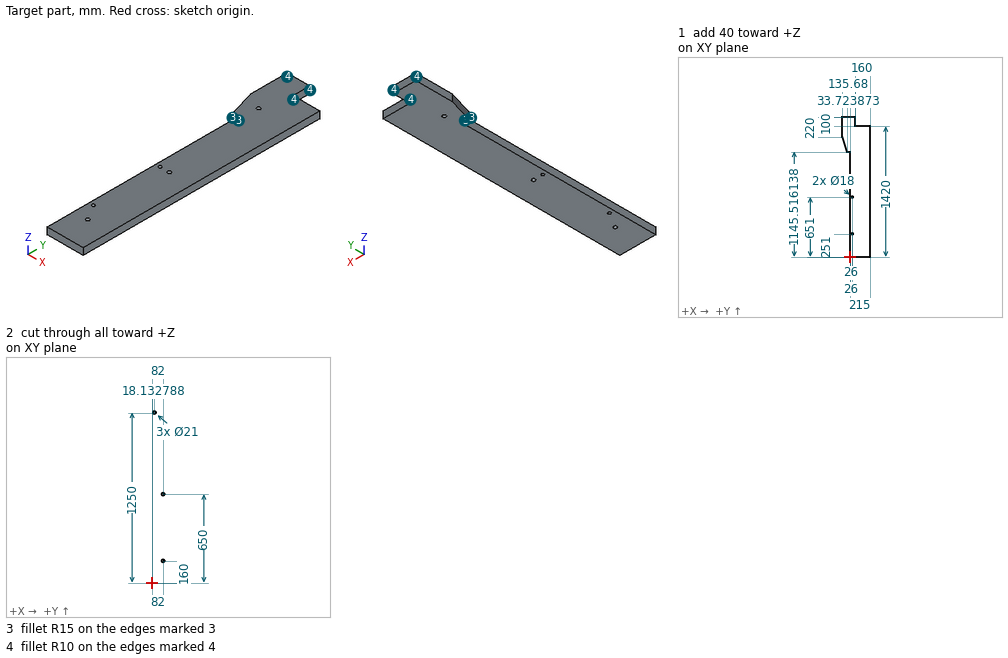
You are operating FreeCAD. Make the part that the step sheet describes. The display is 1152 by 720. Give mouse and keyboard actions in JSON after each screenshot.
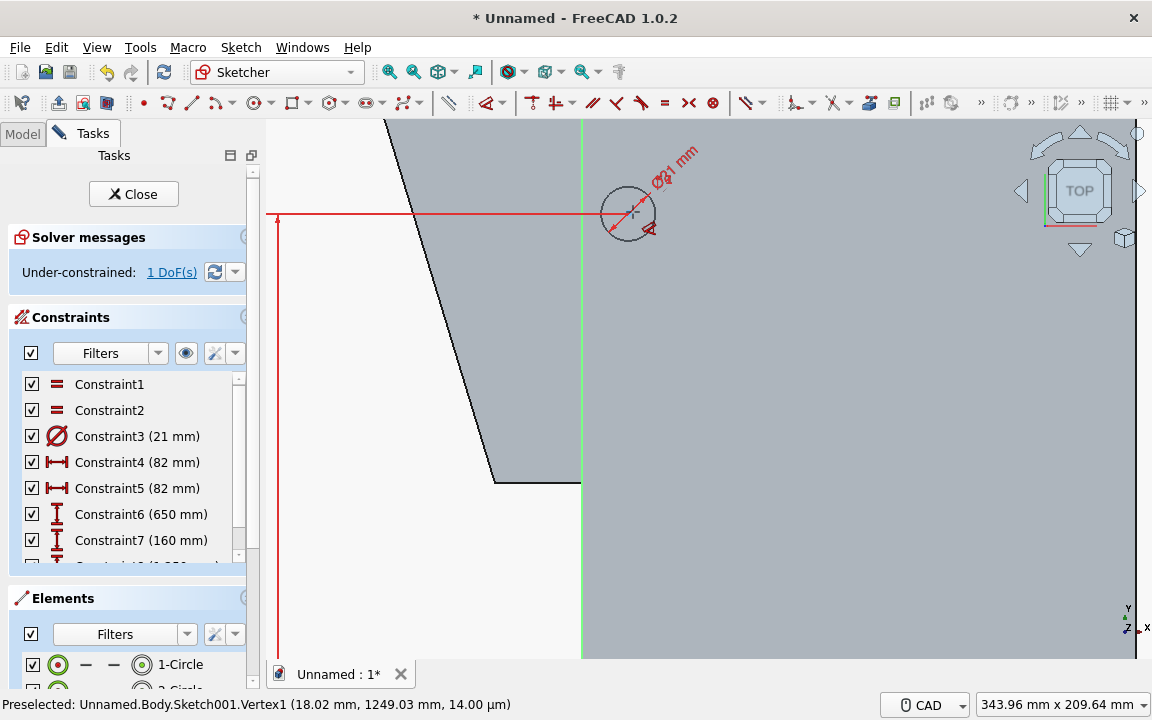
{"action": "left_click", "coordinate": [628, 214]}
{"action": "left_click", "coordinate": [605, 180]}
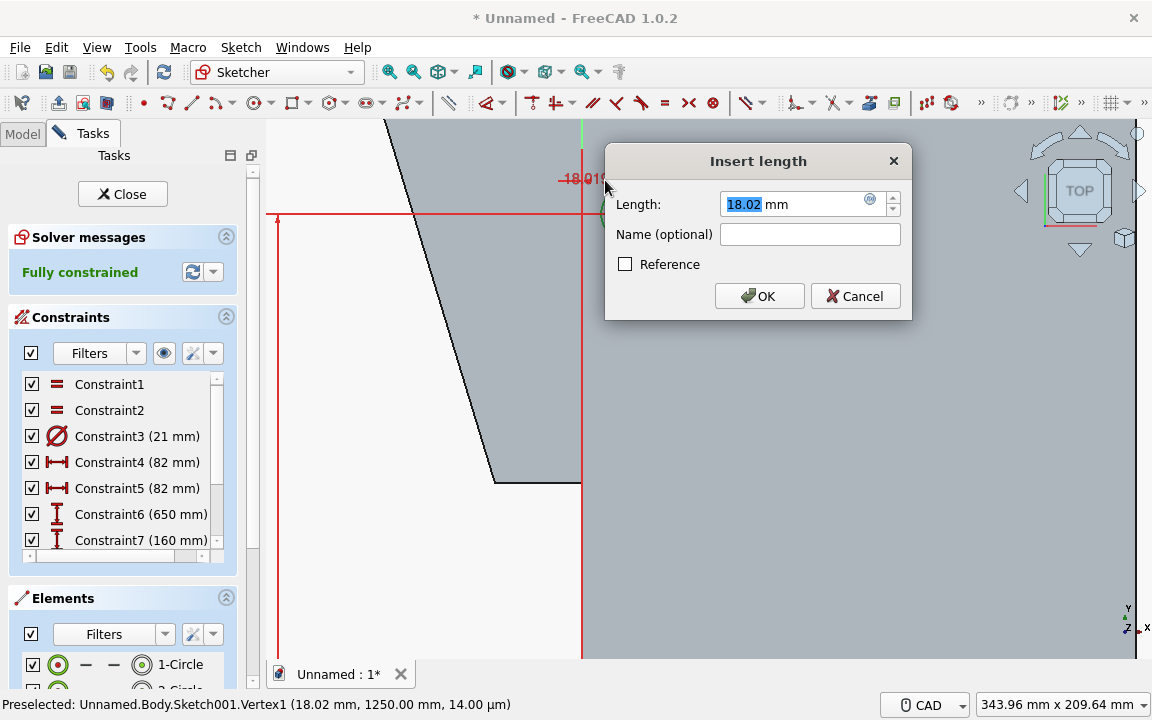
{"action": "type", "text": "18.132788"}
{"action": "key", "text": "Return"}
{"action": "key", "text": "Escape"}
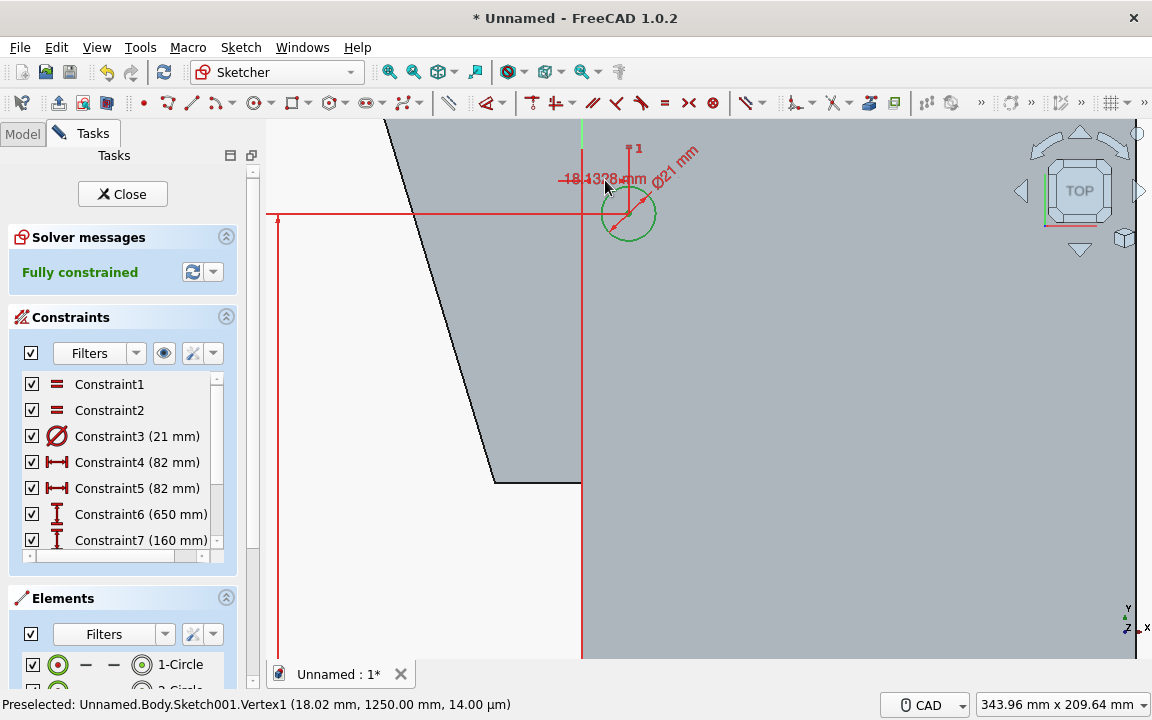
{"action": "left_click", "coordinate": [123, 194]}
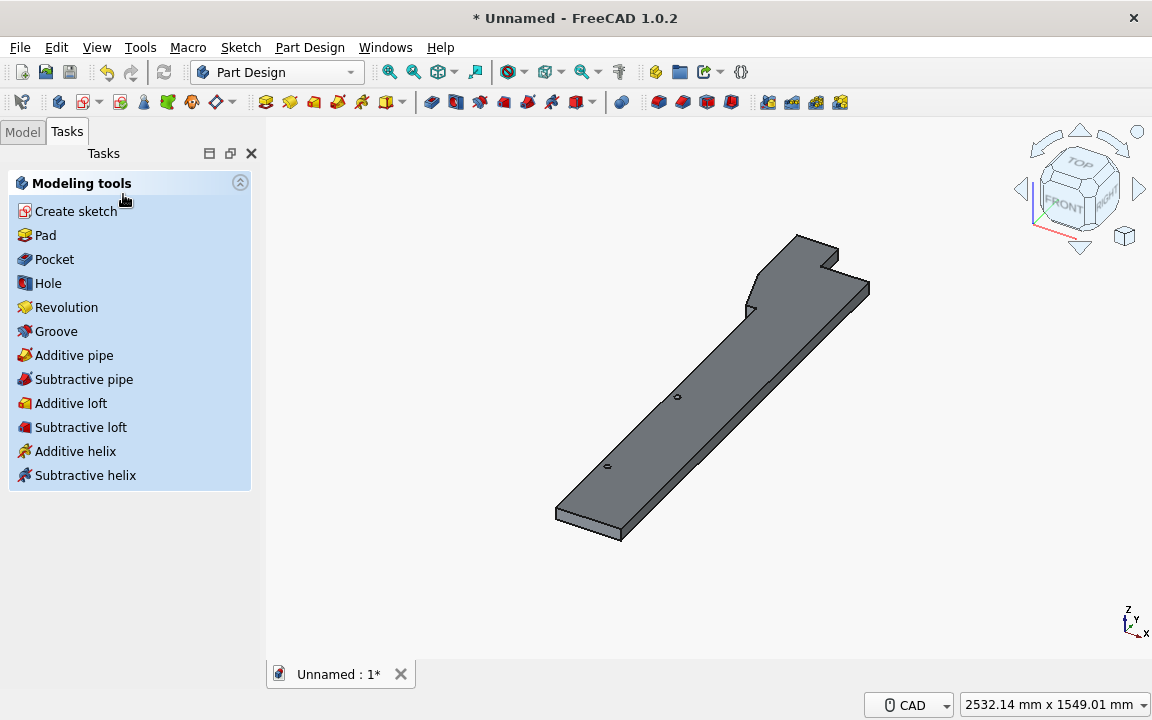
{"action": "left_click", "coordinate": [432, 102]}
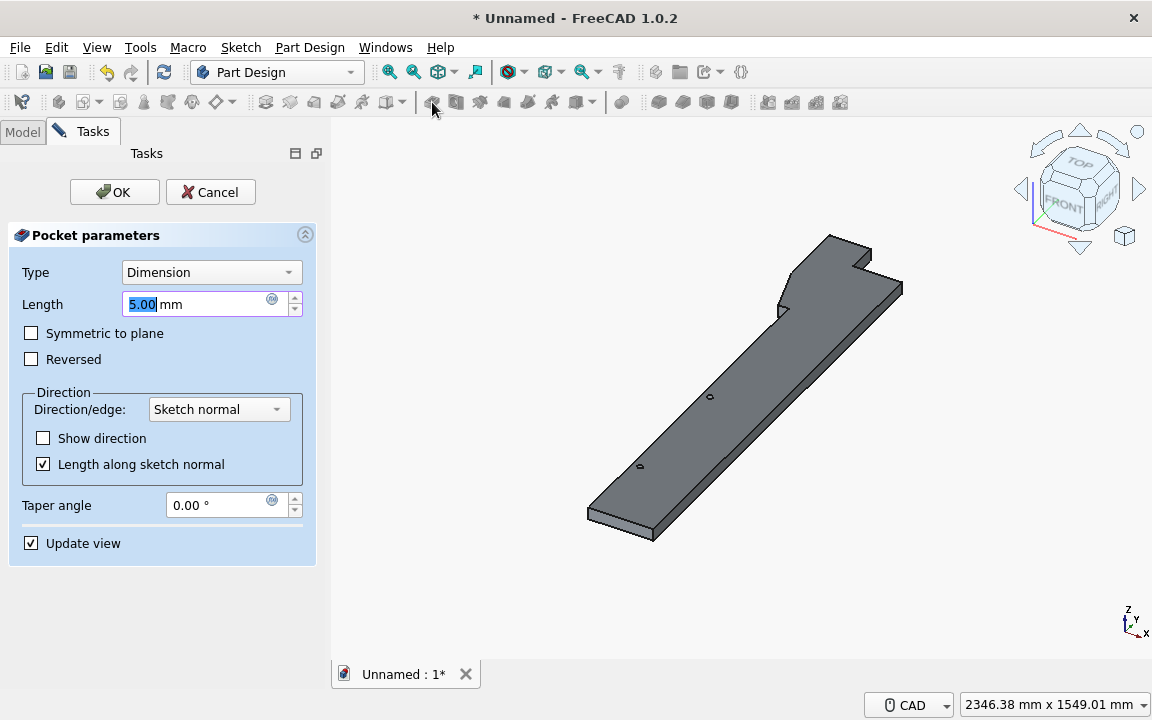
{"action": "left_click", "coordinate": [212, 272]}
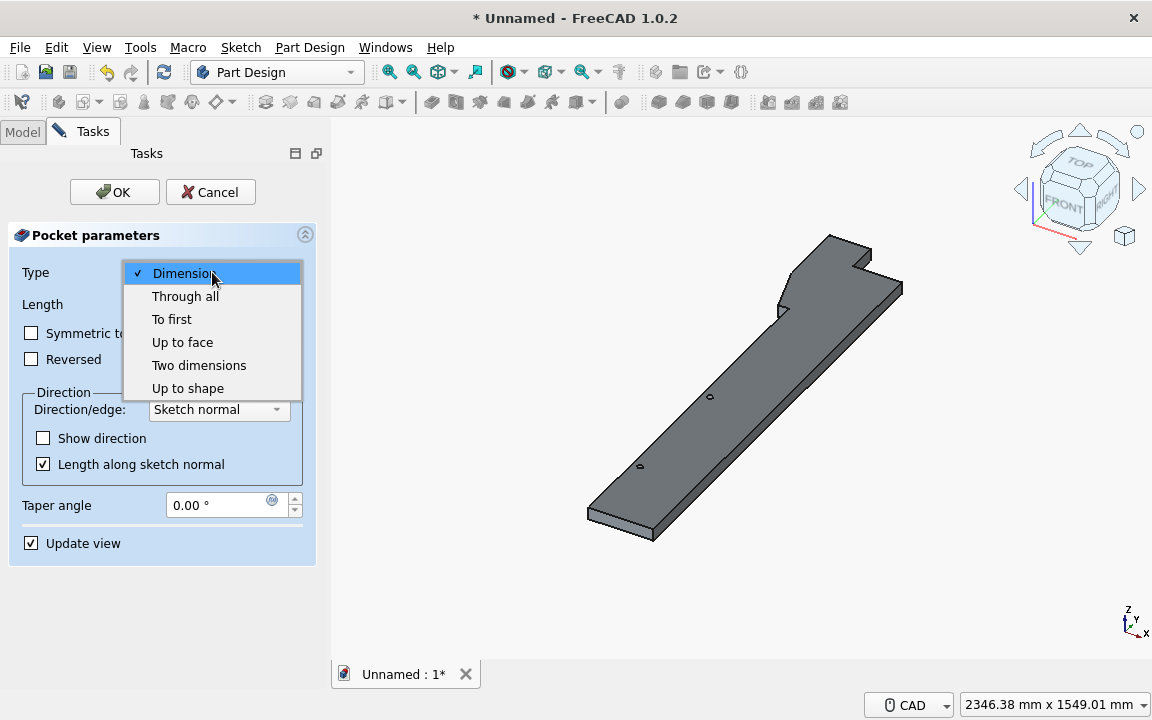
{"action": "left_click", "coordinate": [212, 296]}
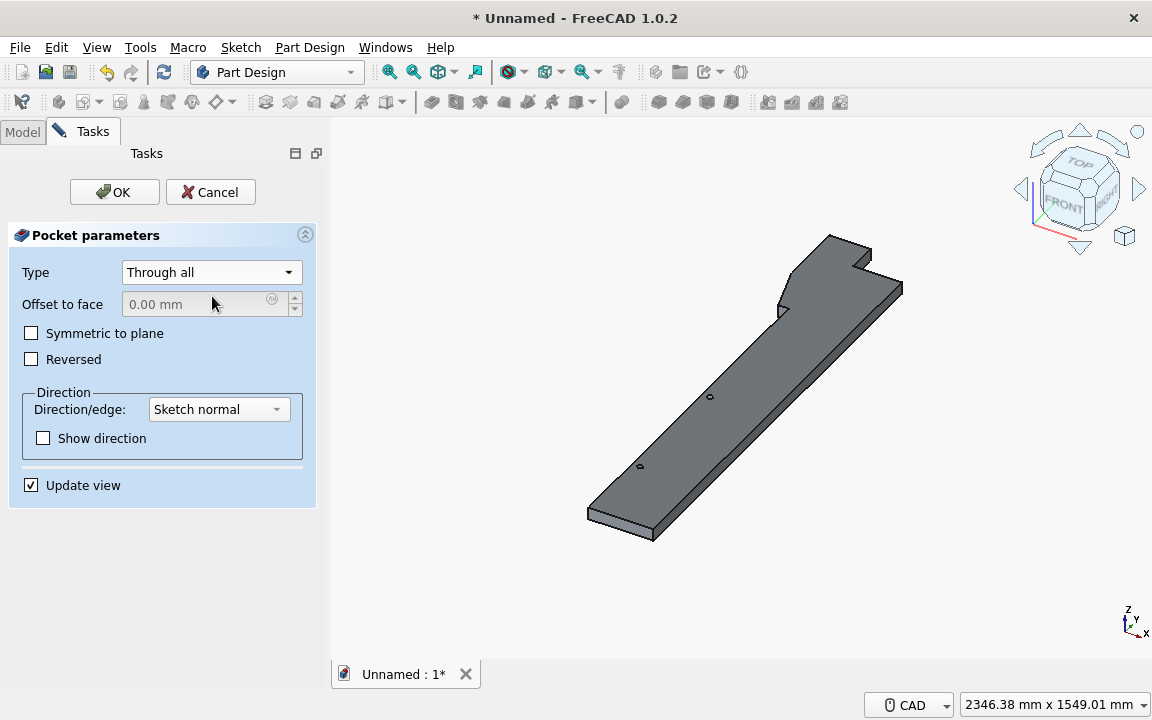
{"action": "left_click", "coordinate": [30, 359]}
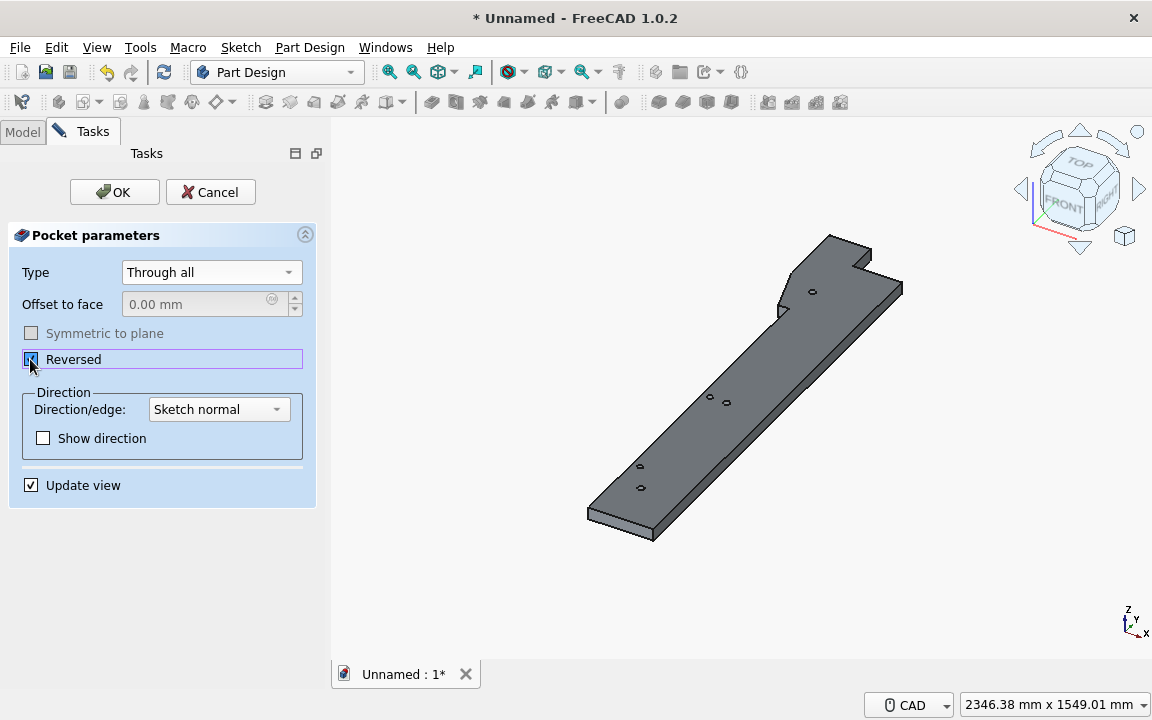
{"action": "left_click", "coordinate": [115, 192]}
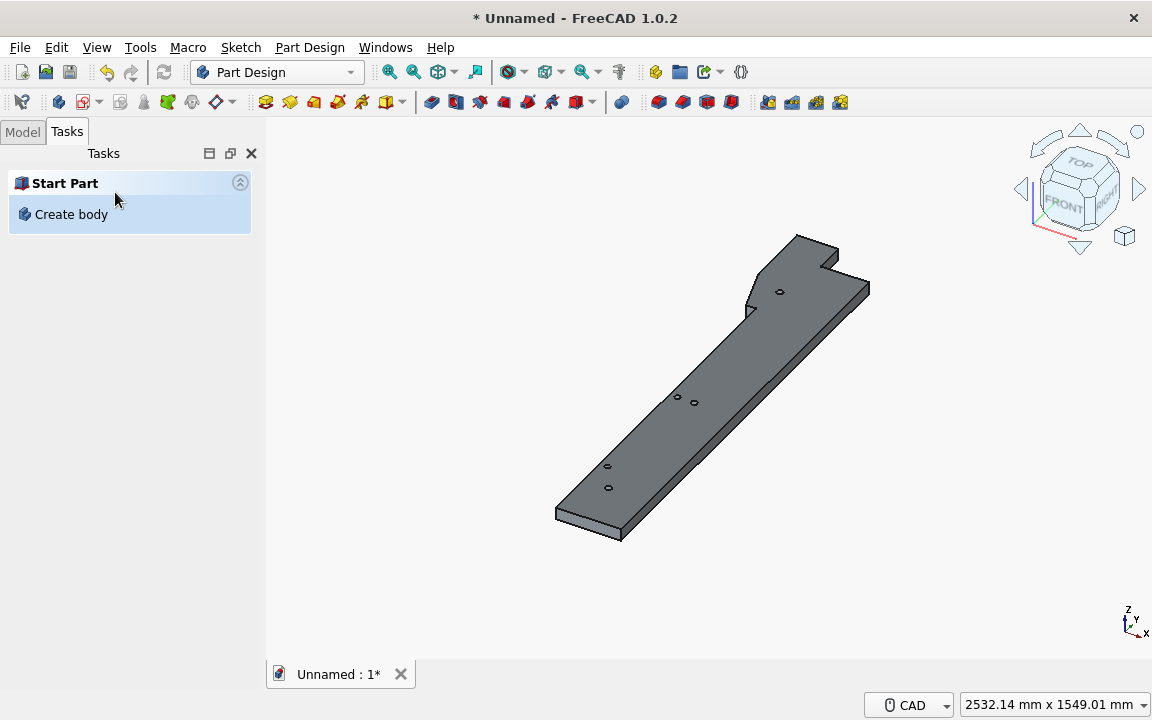
{"action": "scroll", "coordinate": [756, 313], "scroll_direction": "up", "scroll_amount": 6}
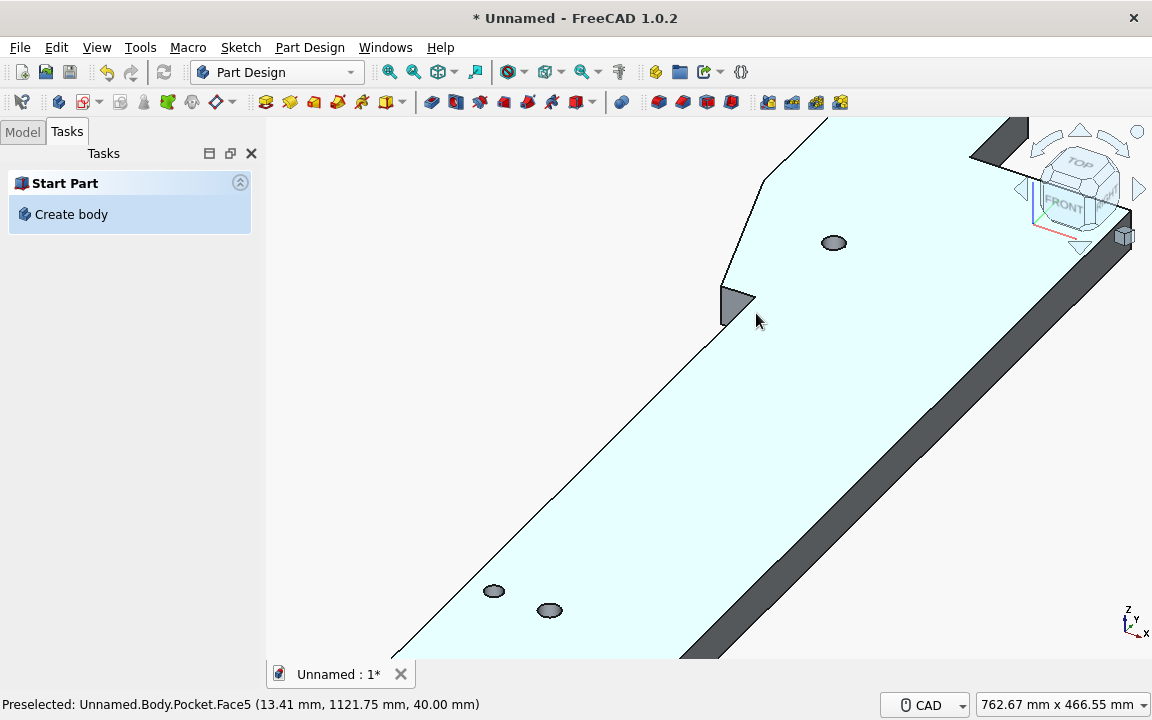
{"action": "left_click", "coordinate": [390, 72]}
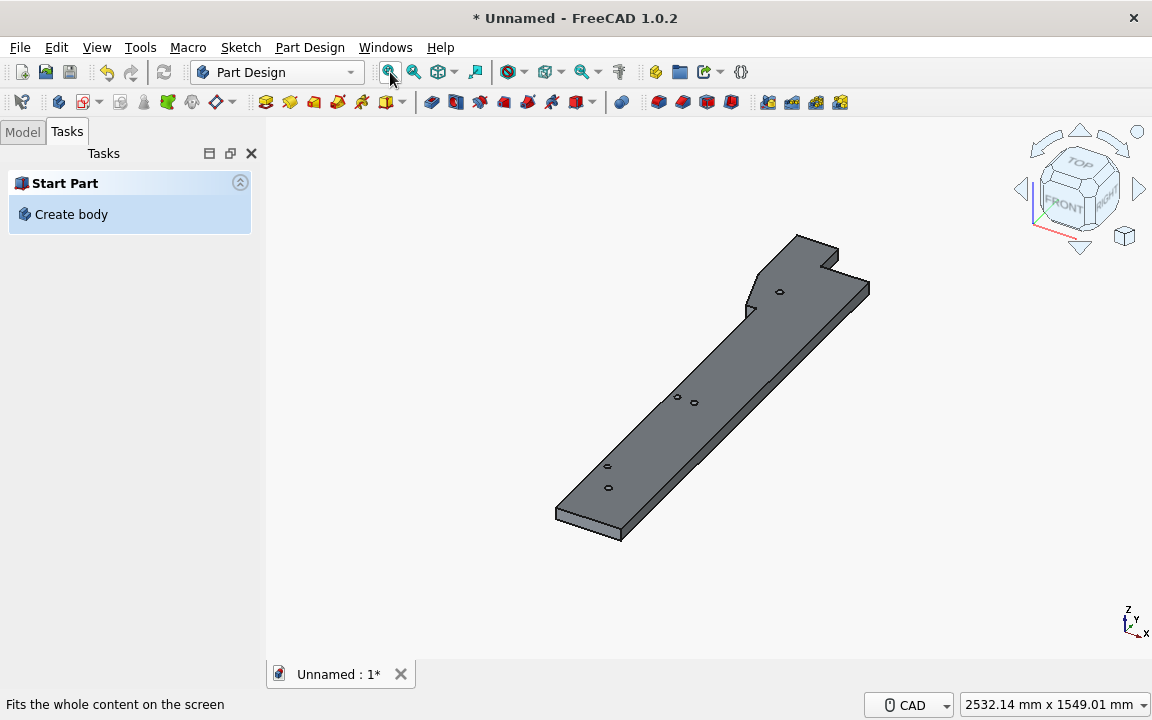
{"action": "key", "text": "0"}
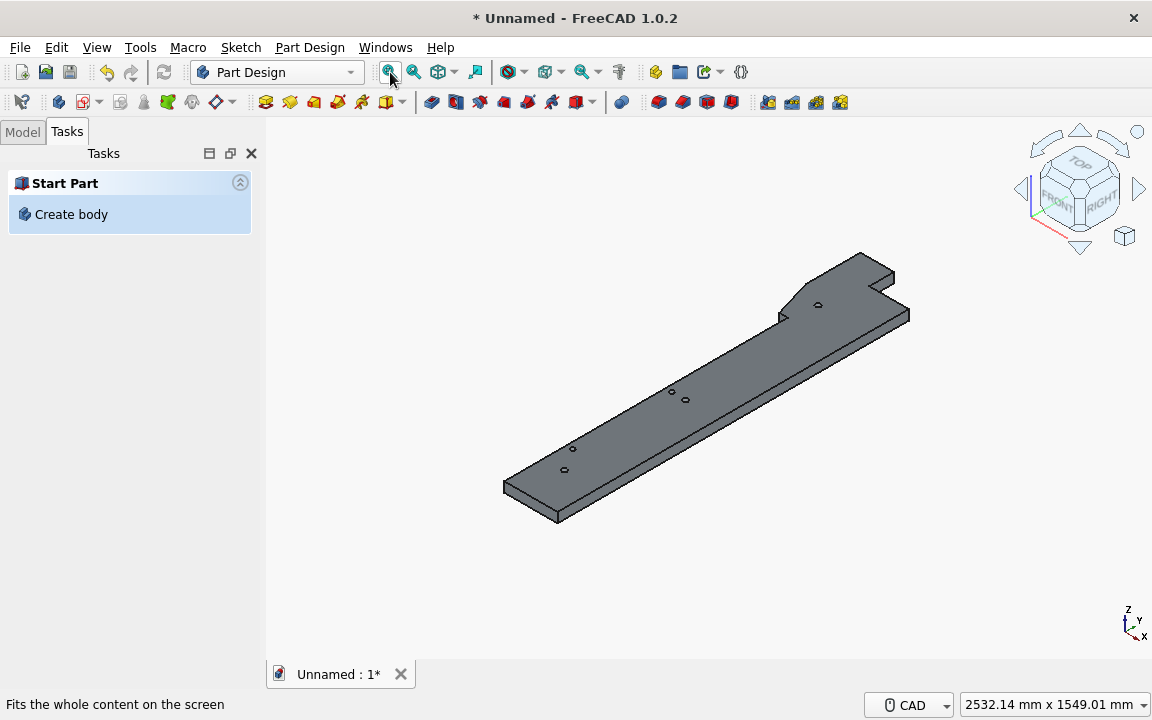
{"action": "scroll", "coordinate": [788, 322], "scroll_direction": "up", "scroll_amount": 6}